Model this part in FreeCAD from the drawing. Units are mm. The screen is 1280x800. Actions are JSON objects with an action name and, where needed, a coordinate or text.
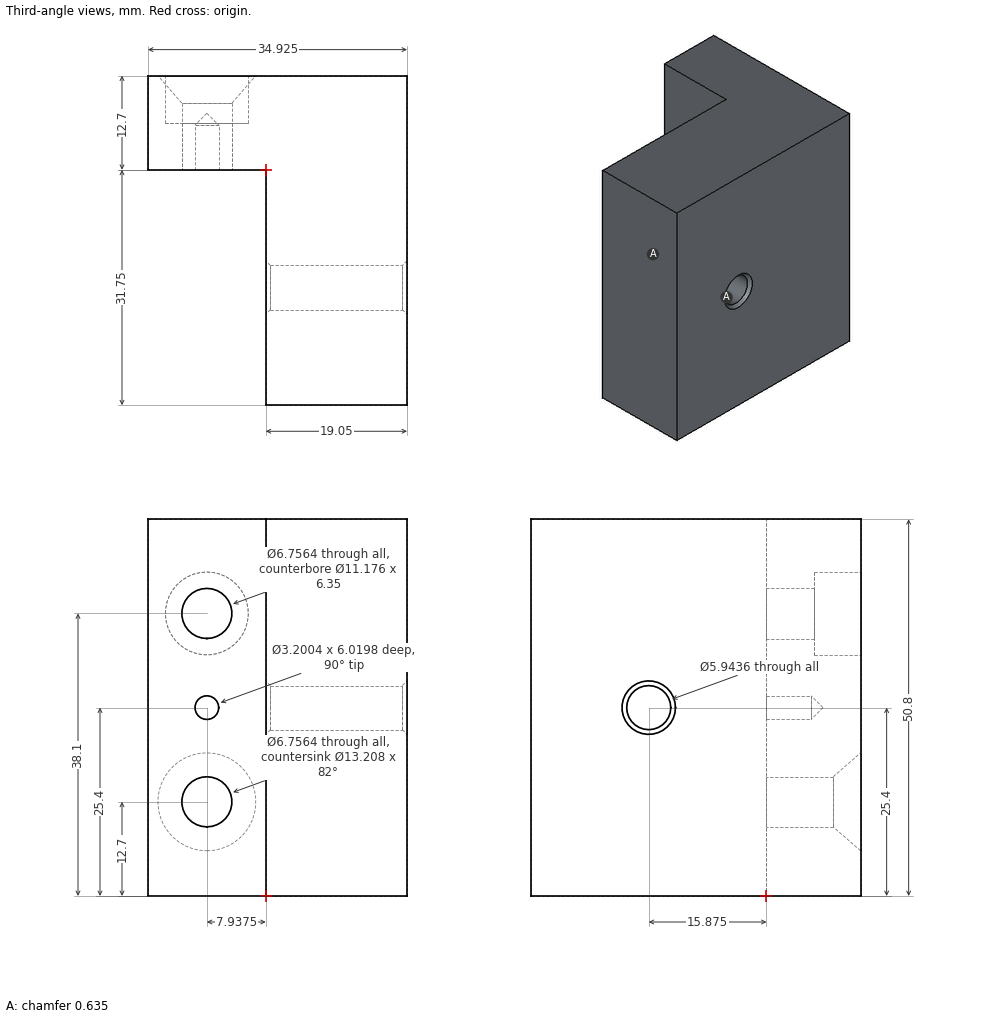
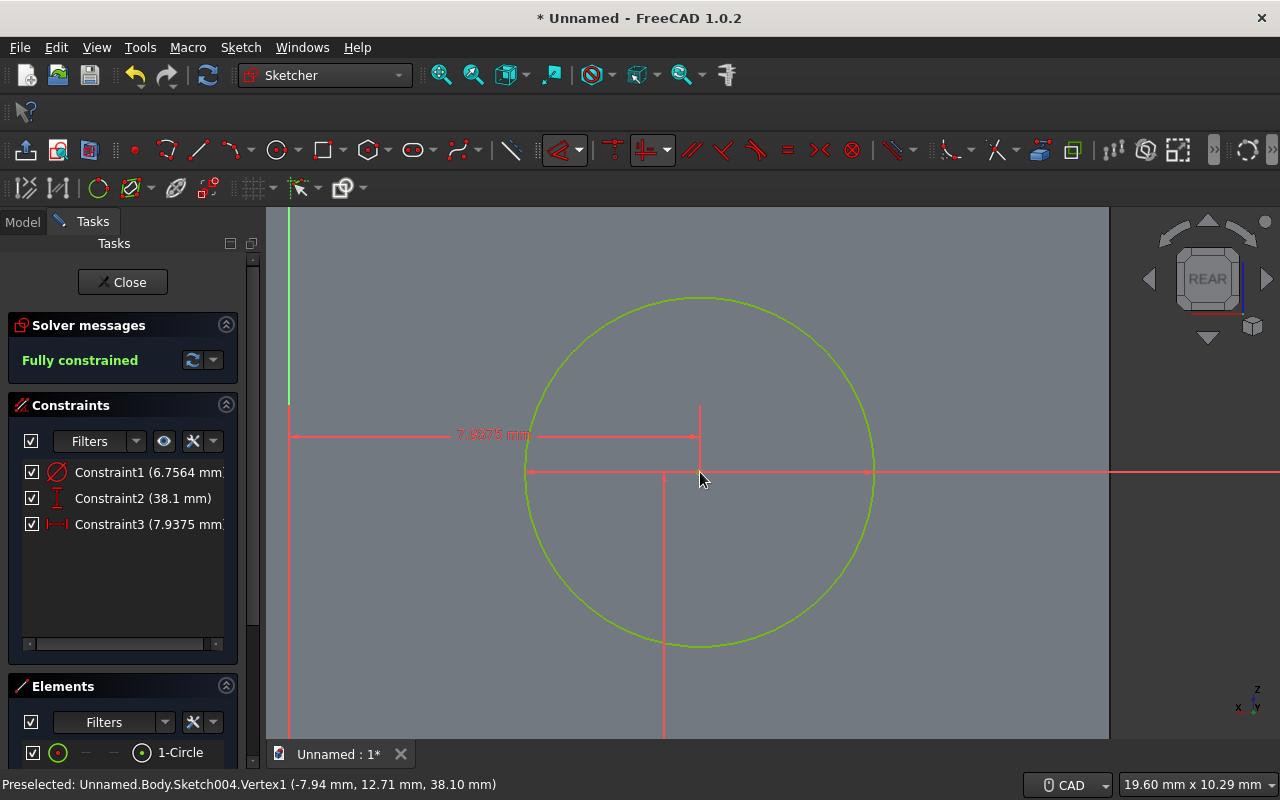
{"action": "left_click", "coordinate": [123, 282]}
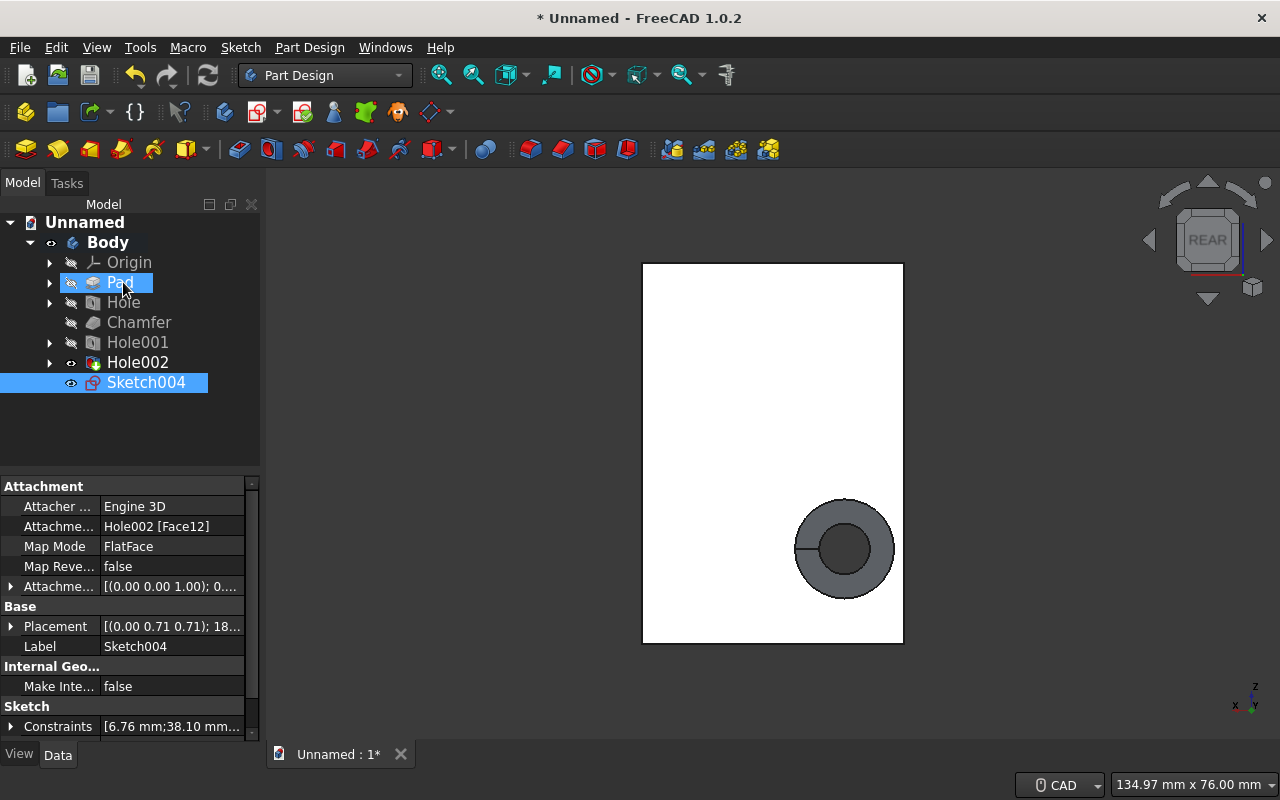
{"action": "left_click", "coordinate": [272, 150]}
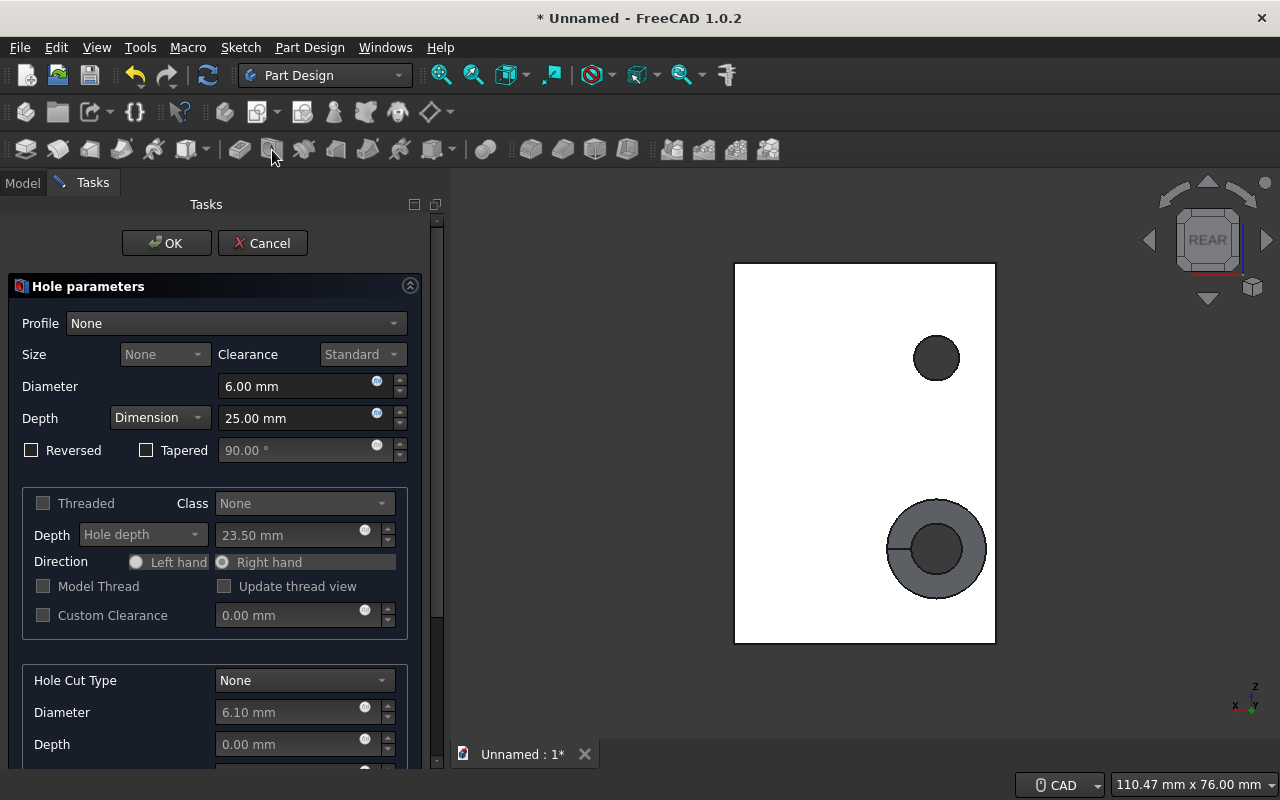
{"action": "triple_click", "coordinate": [305, 386]}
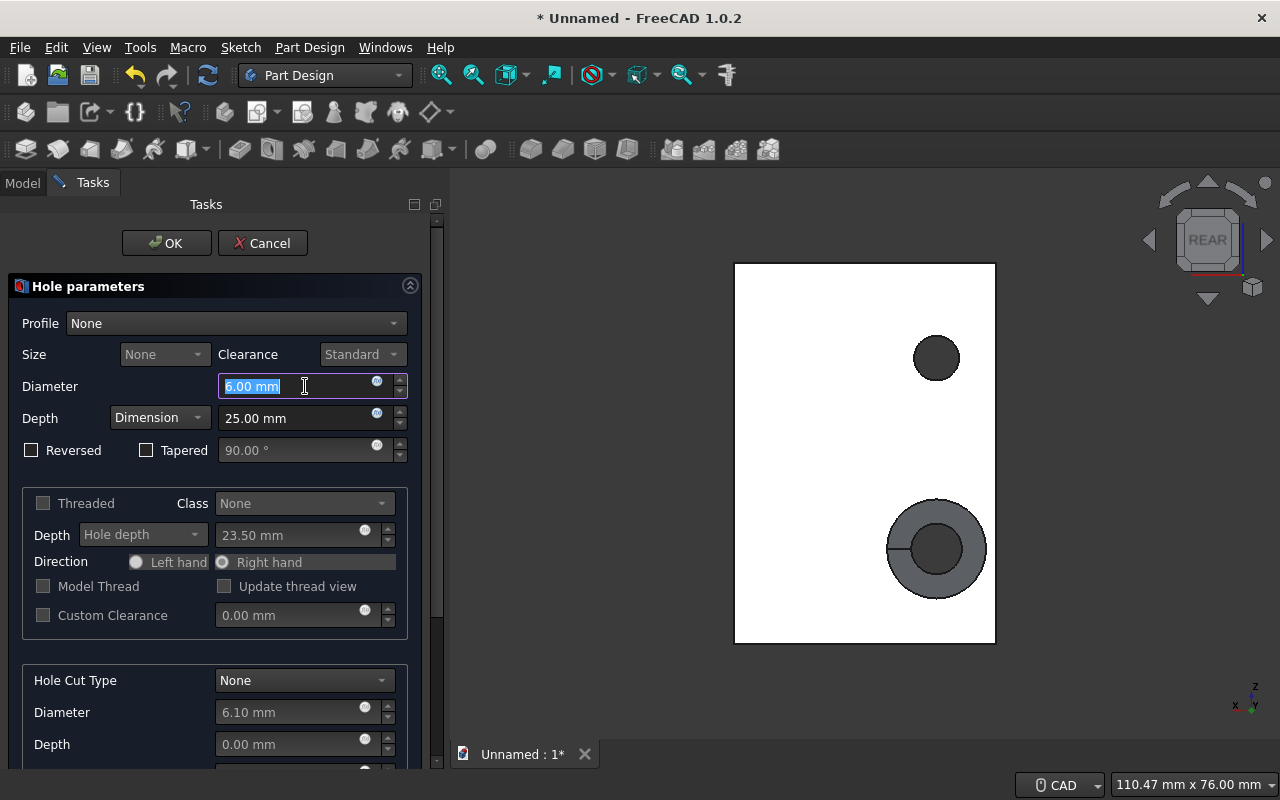
{"action": "type", "text": "6.7564"}
{"action": "key", "text": "Tab"}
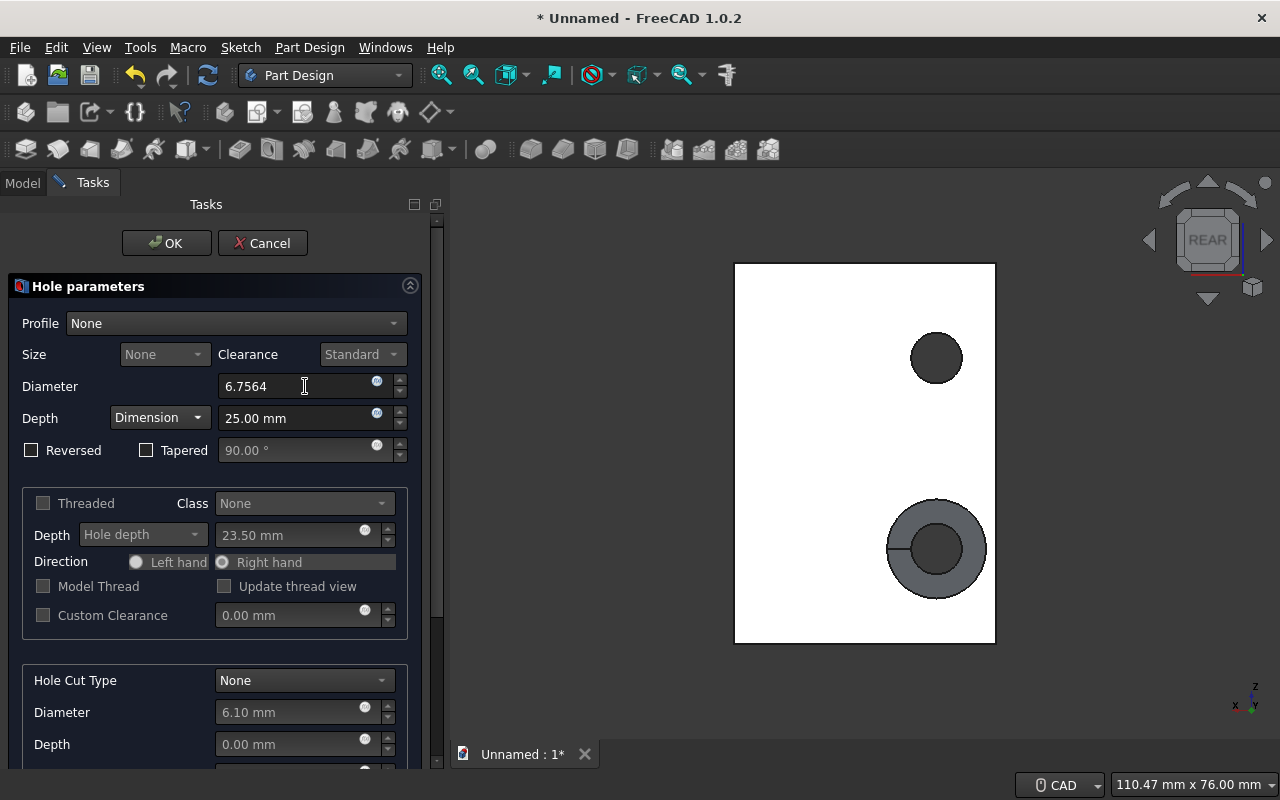
{"action": "left_click", "coordinate": [161, 418]}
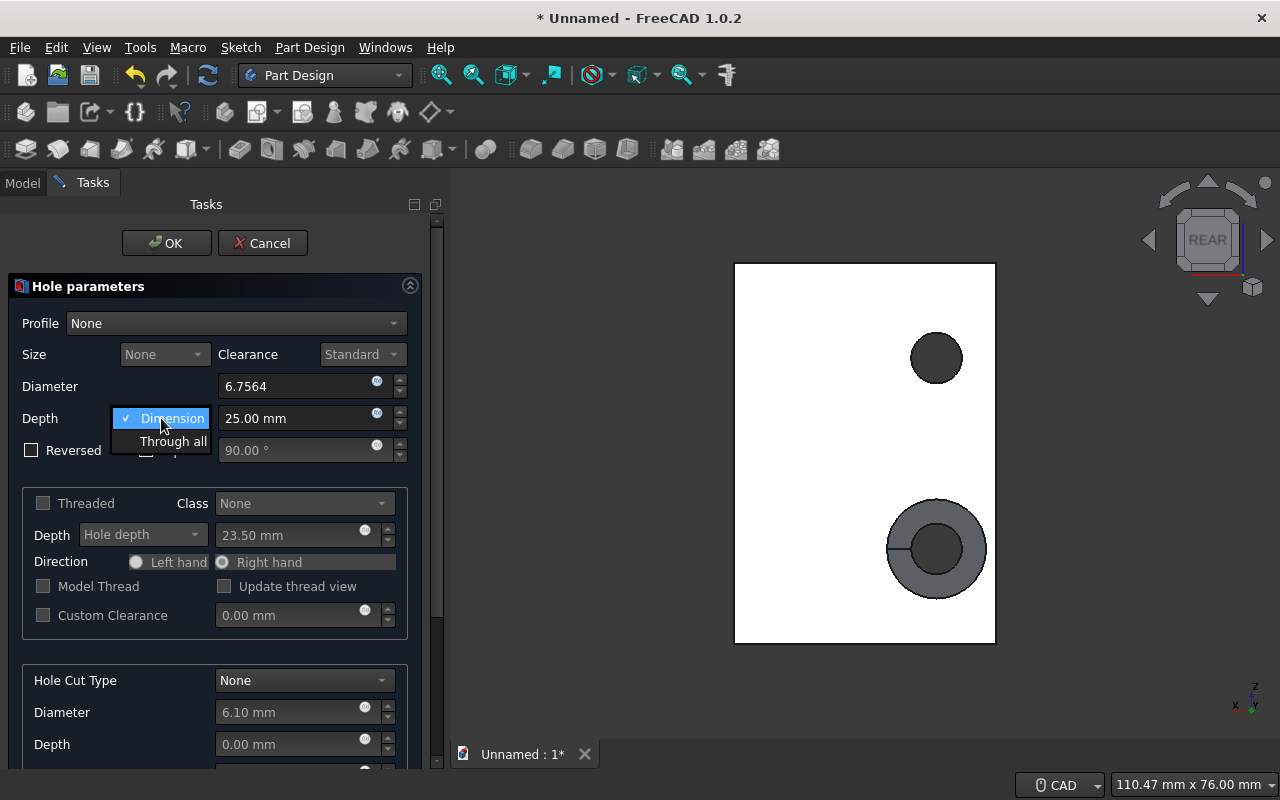
{"action": "left_click", "coordinate": [160, 442]}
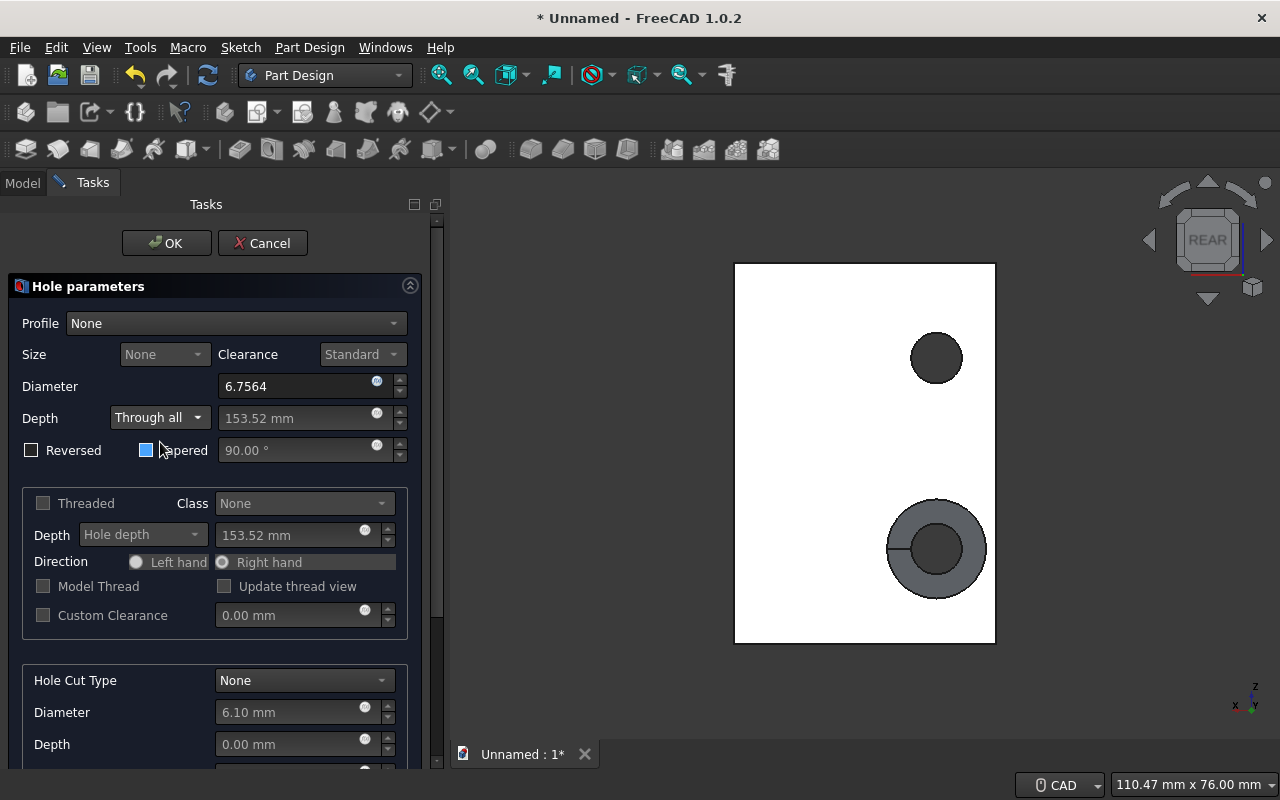
{"action": "left_click", "coordinate": [306, 680]}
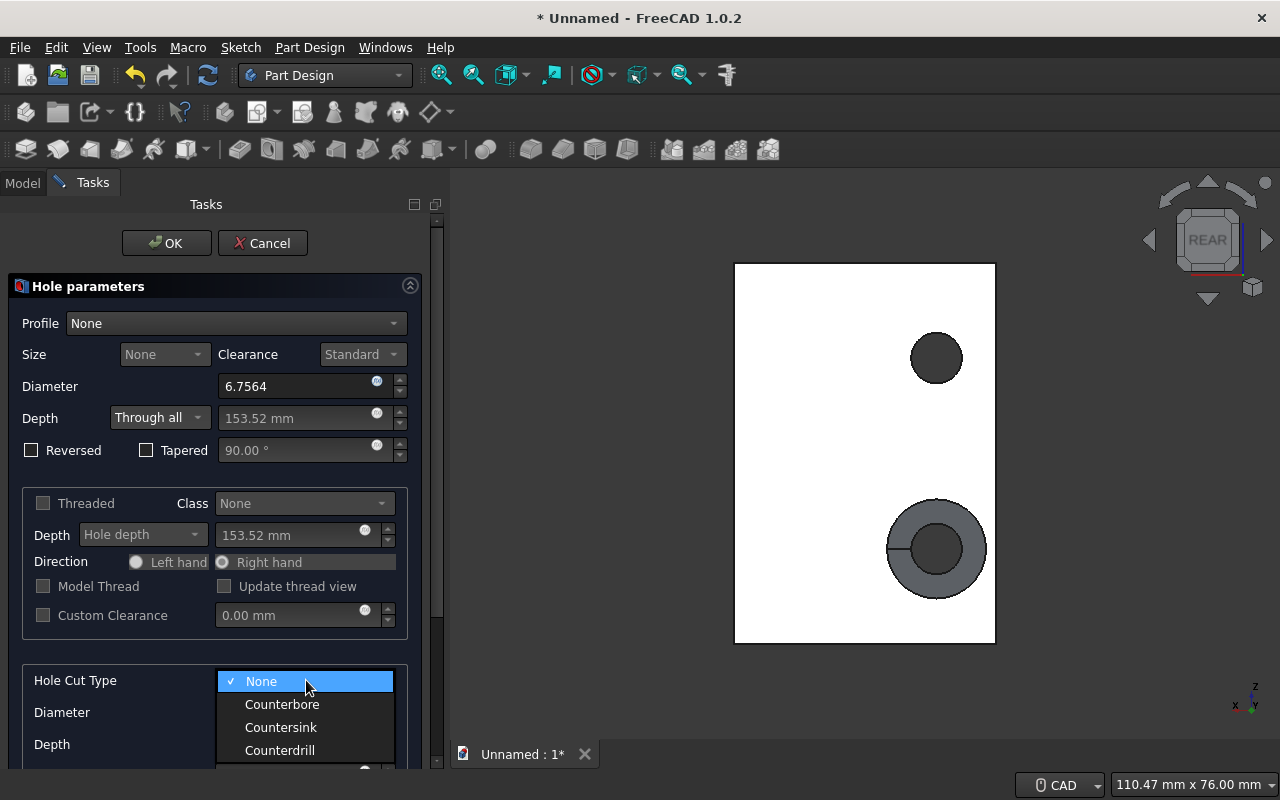
{"action": "left_click", "coordinate": [304, 704]}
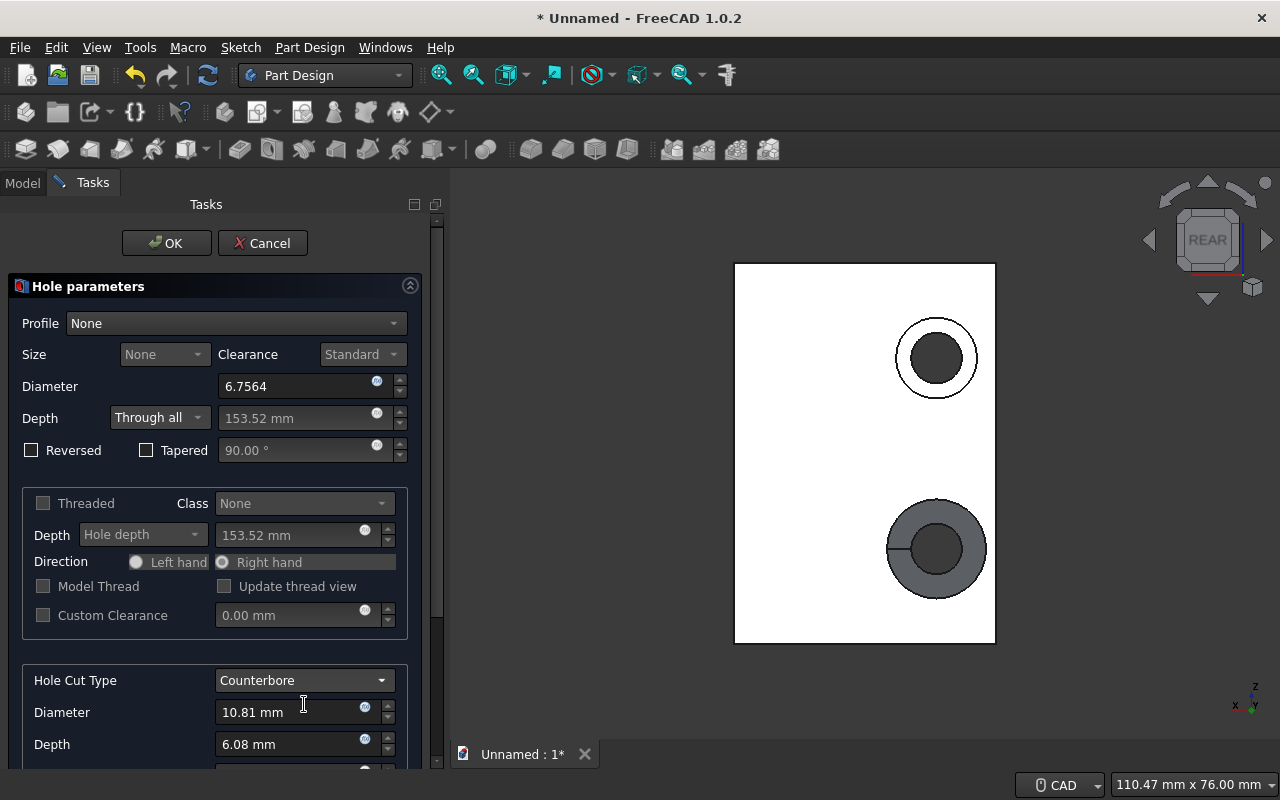
{"action": "triple_click", "coordinate": [298, 712]}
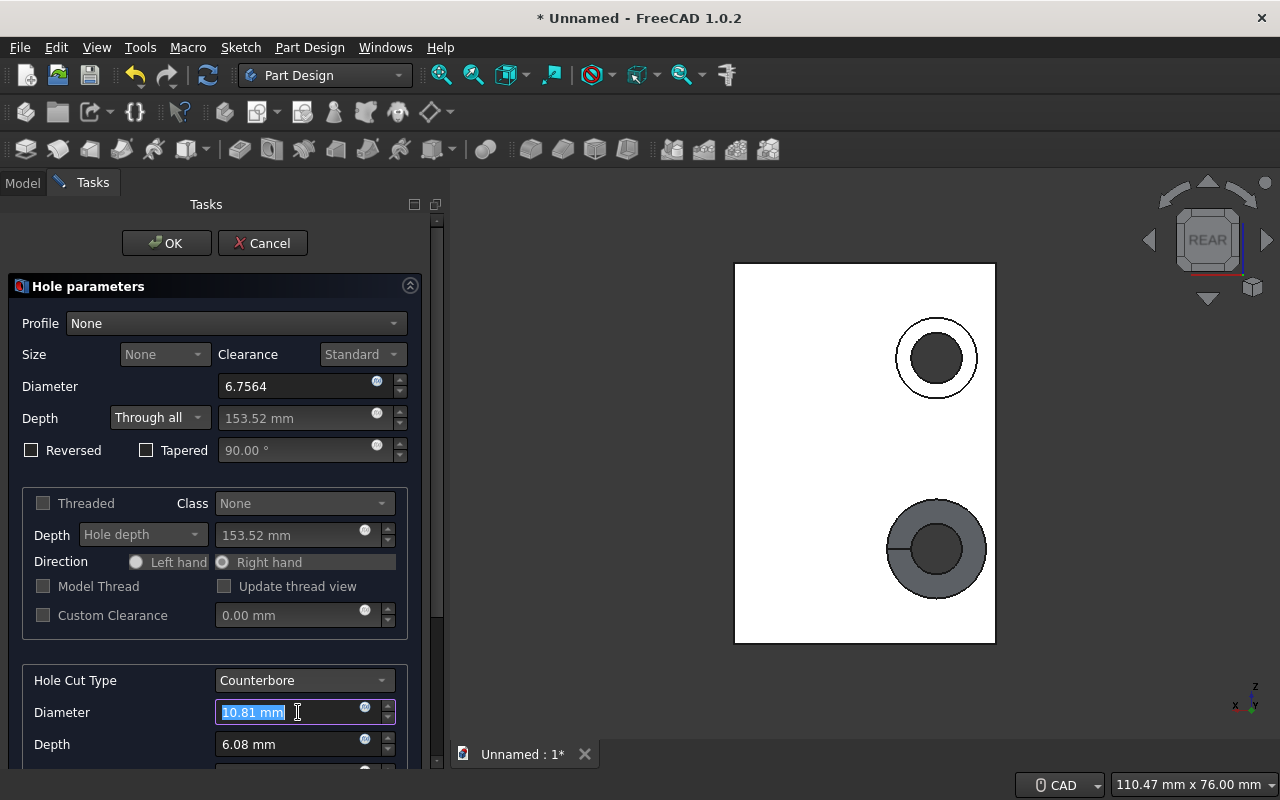
{"action": "type", "text": "11.176"}
{"action": "key", "text": "Tab"}